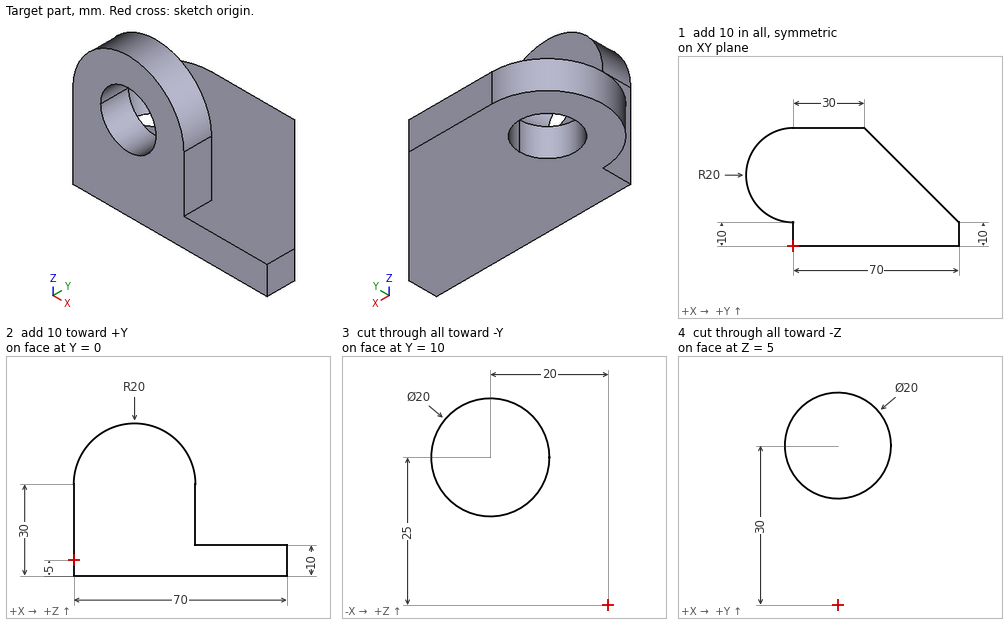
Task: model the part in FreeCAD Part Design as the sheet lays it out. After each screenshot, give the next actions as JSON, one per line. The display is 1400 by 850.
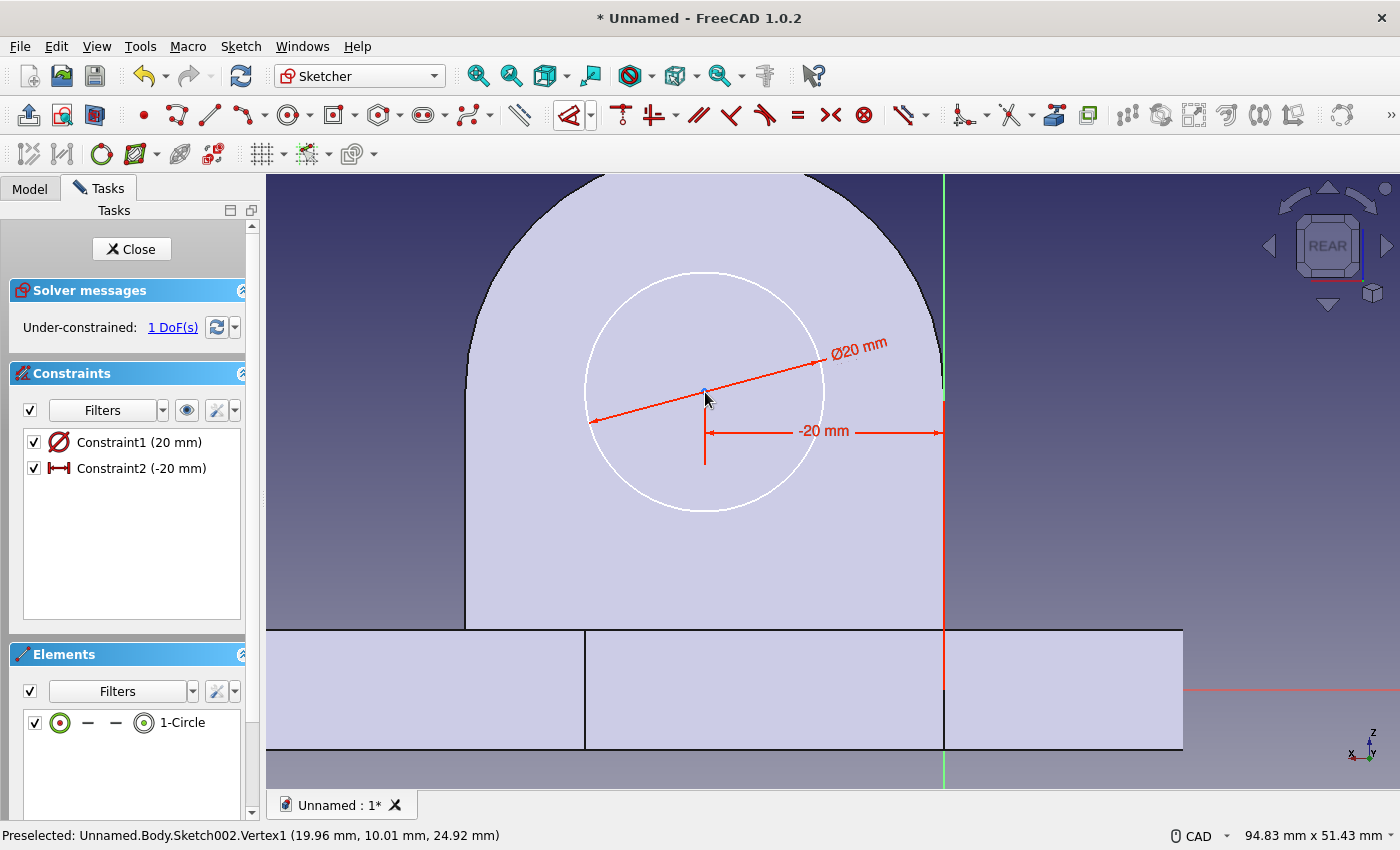
{"action": "left_click", "coordinate": [705, 392]}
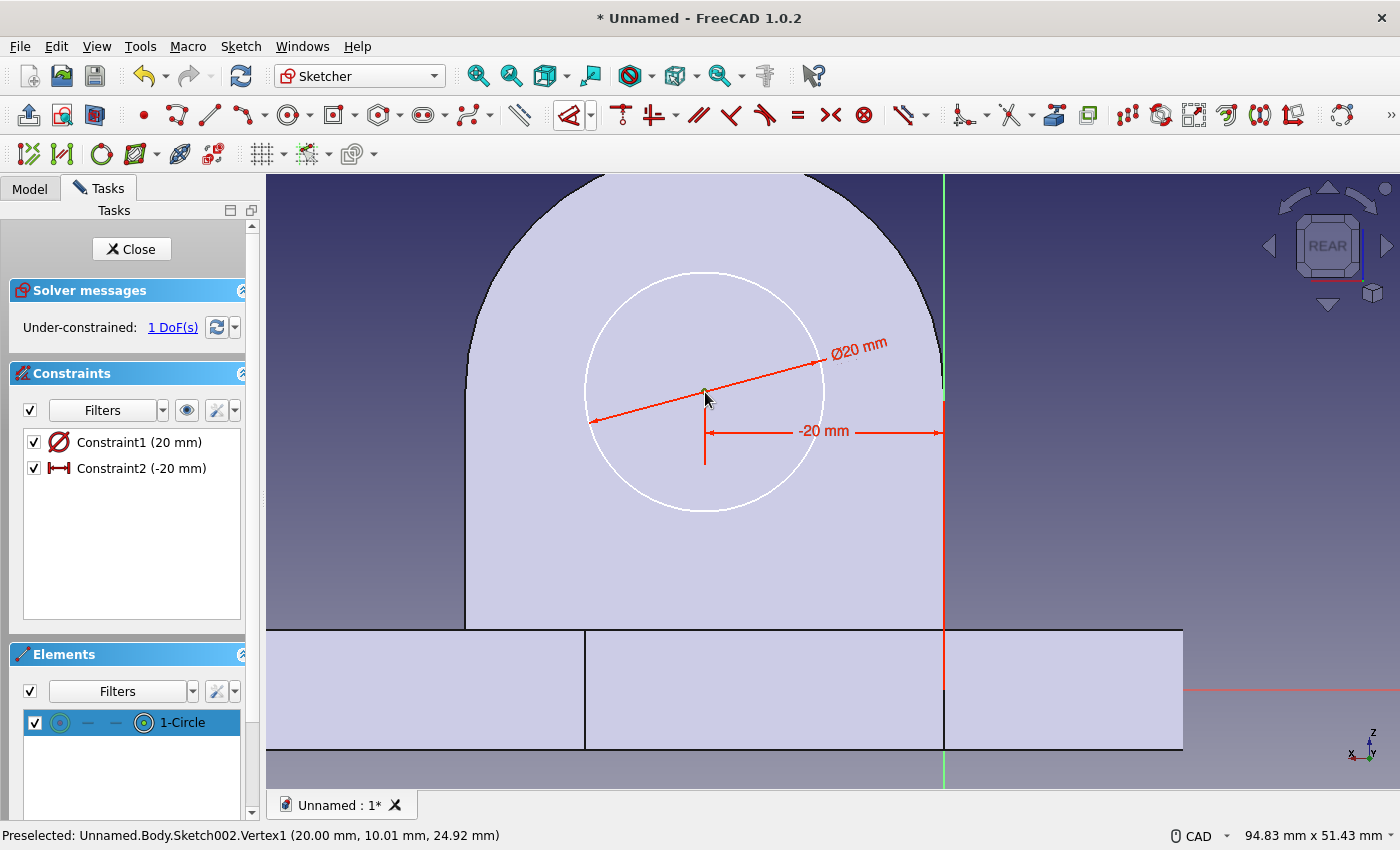
{"action": "key", "text": "i"}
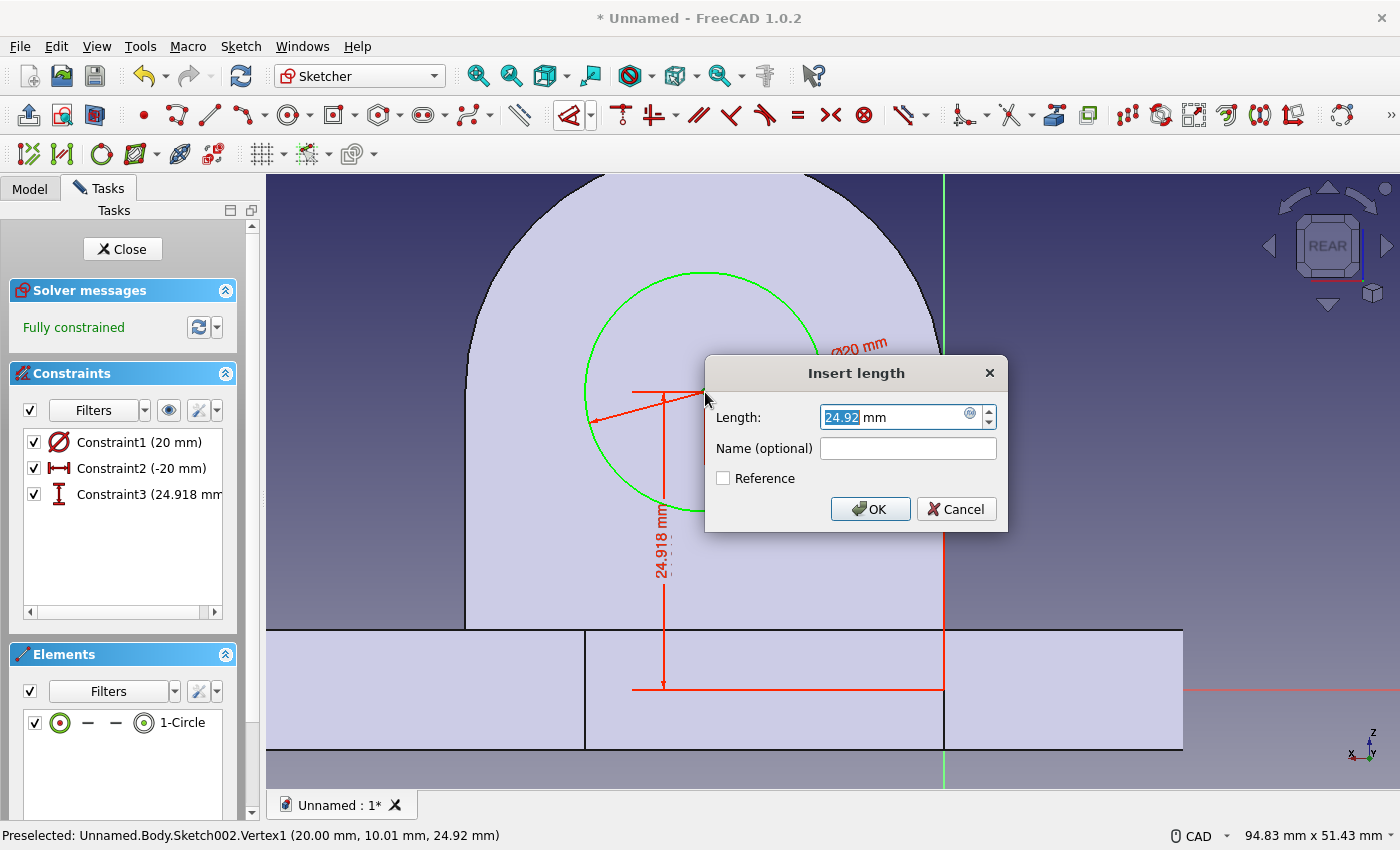
{"action": "type", "text": "25"}
{"action": "key", "text": "Return"}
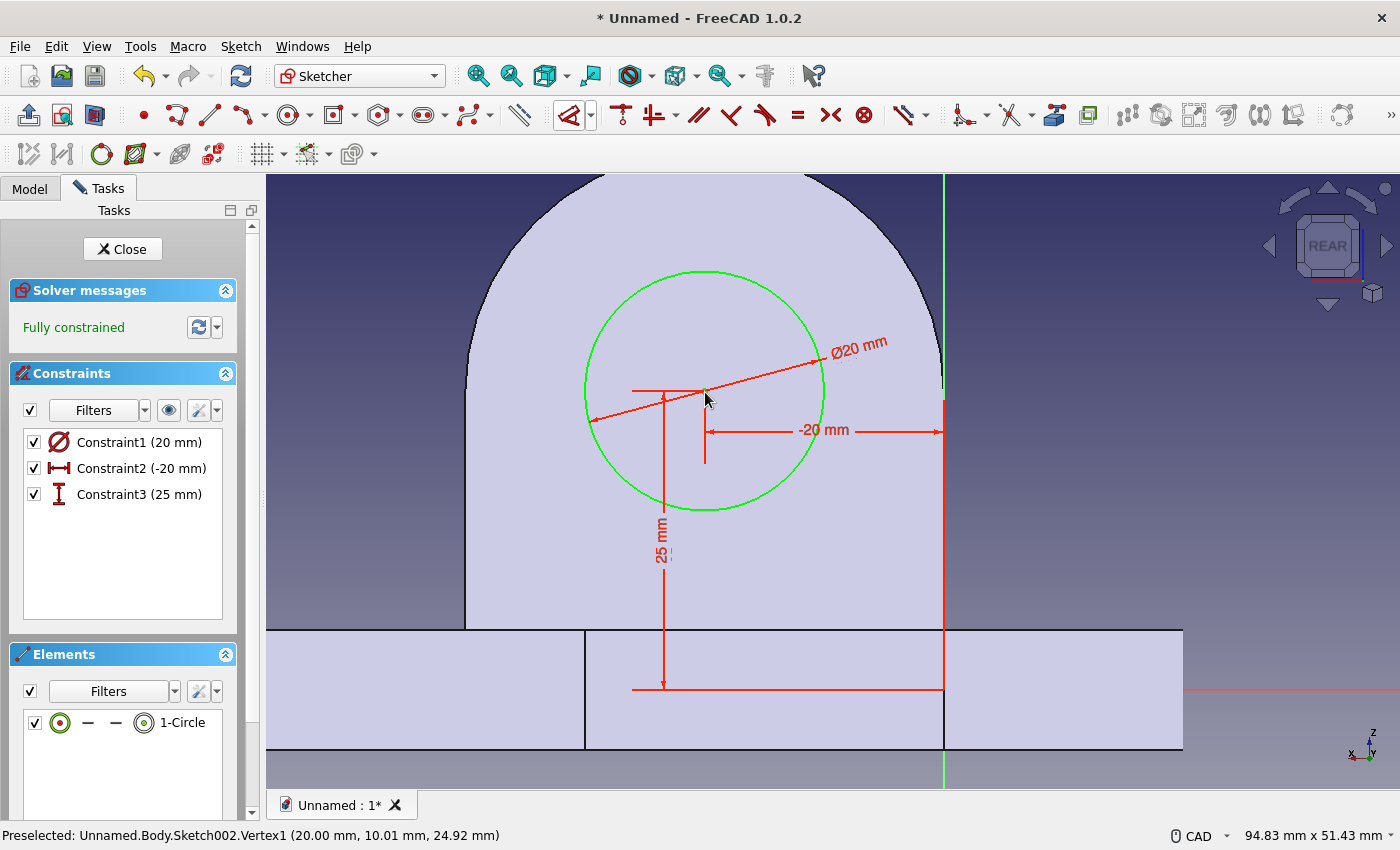
{"action": "left_click", "coordinate": [123, 249]}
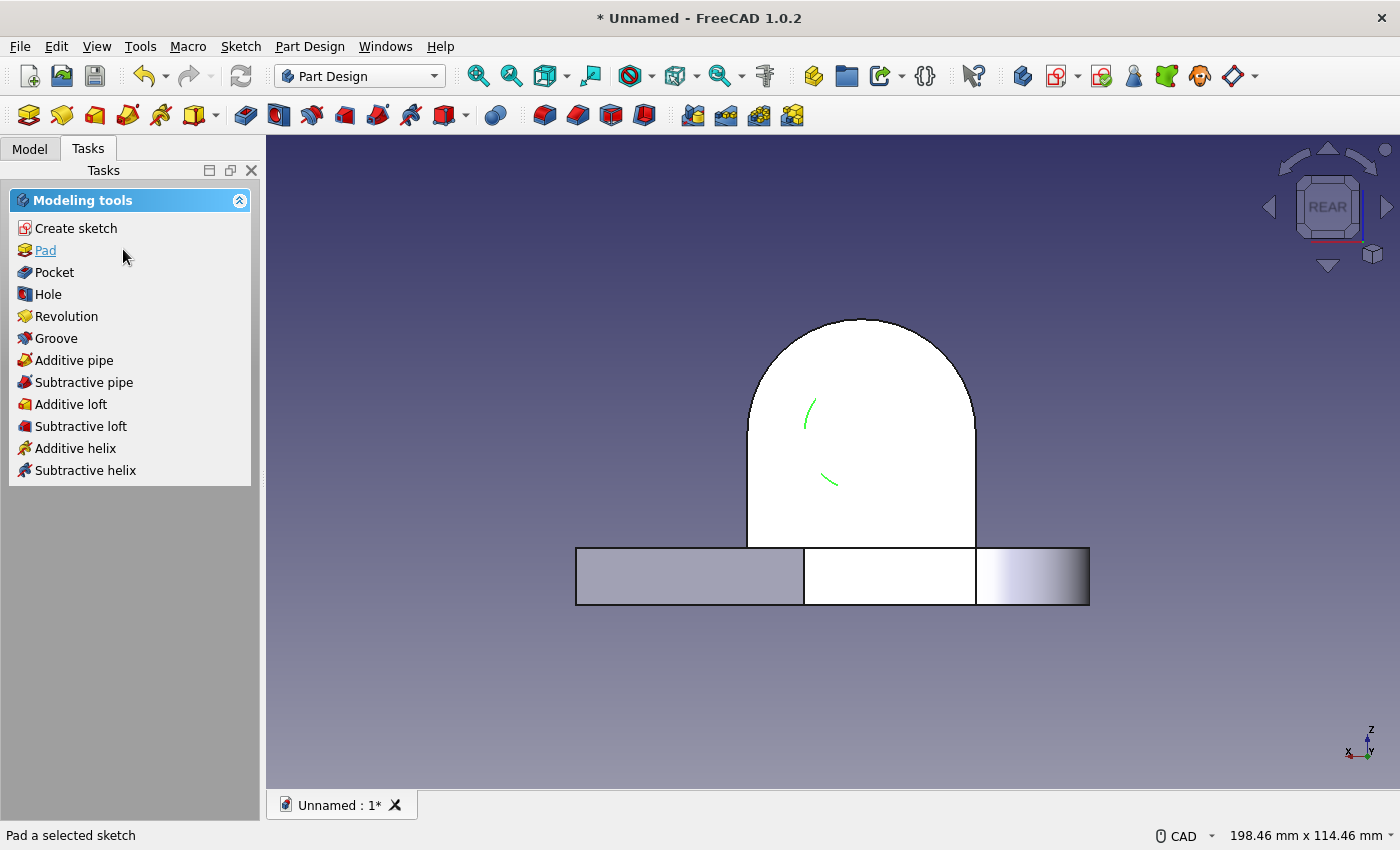
{"action": "left_click", "coordinate": [246, 116]}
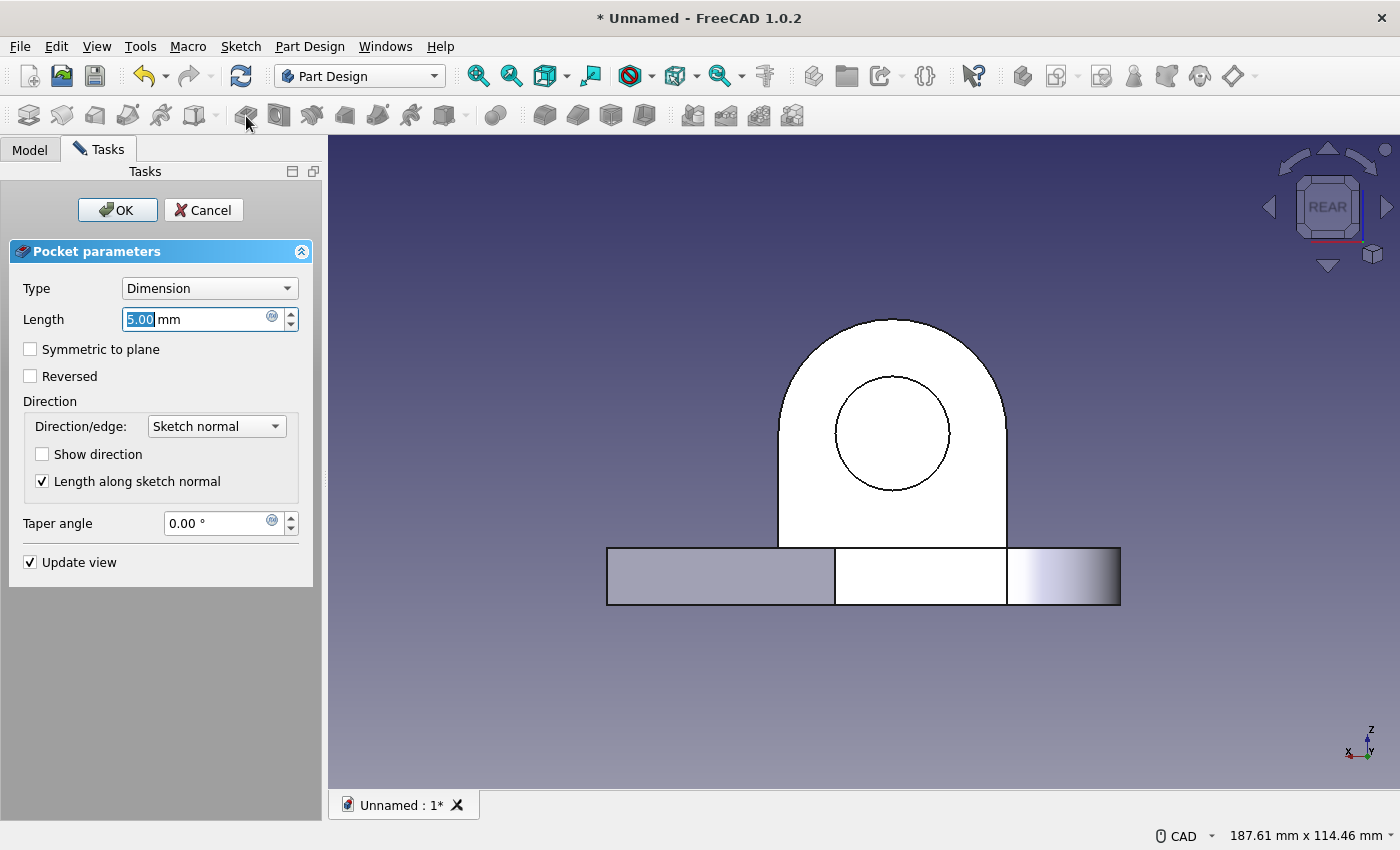
{"action": "left_click", "coordinate": [210, 288]}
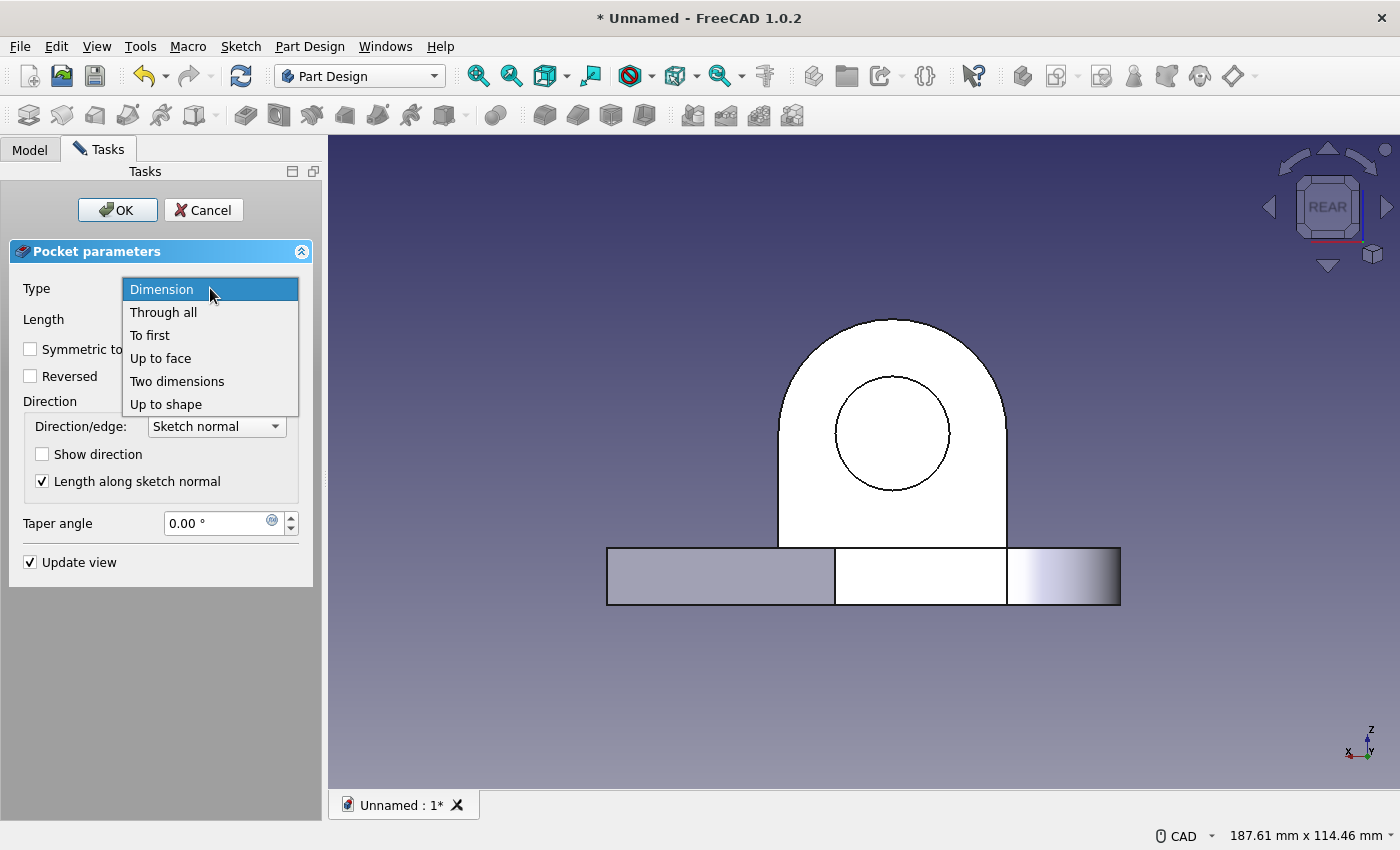
{"action": "left_click", "coordinate": [208, 312]}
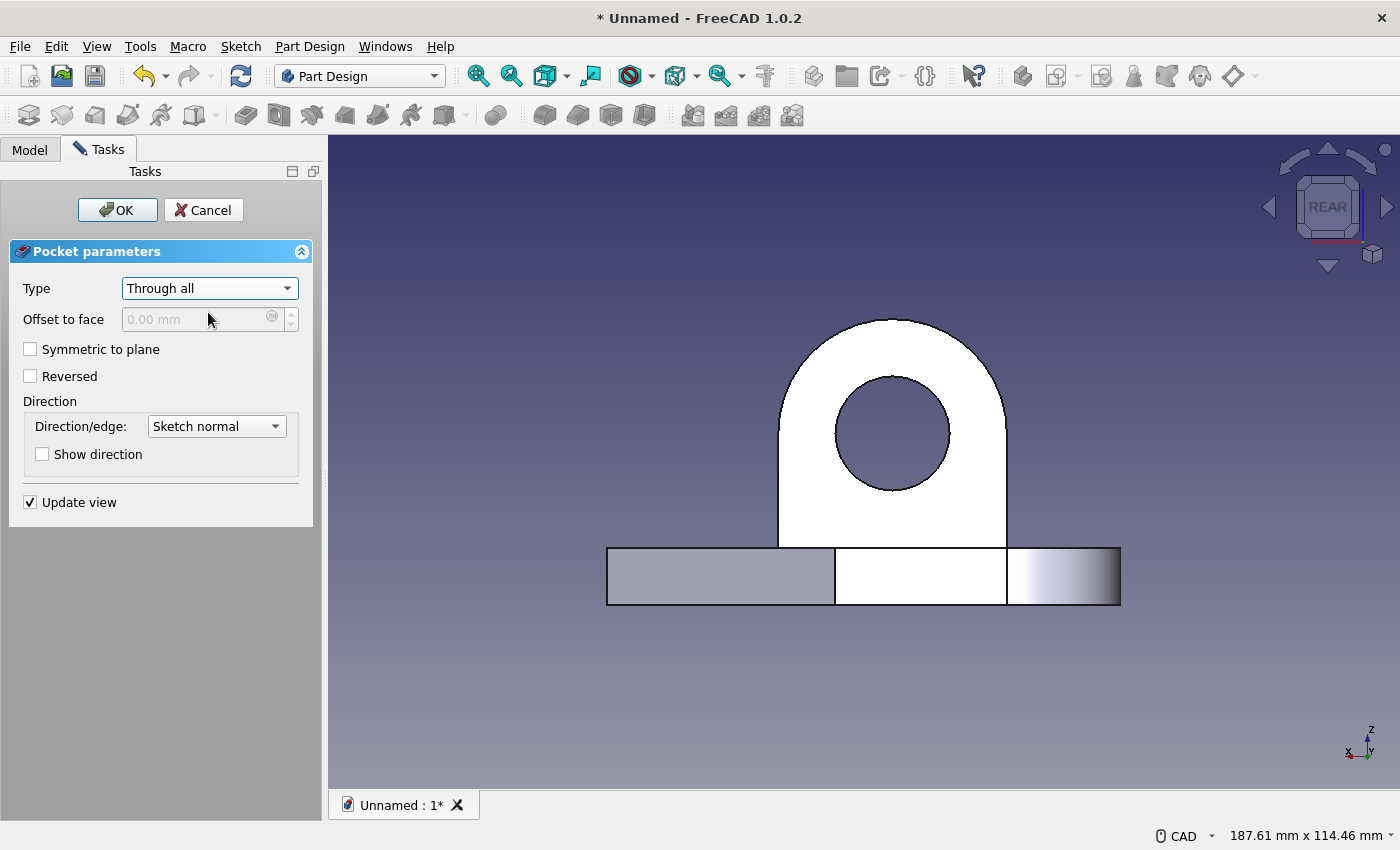
{"action": "left_click", "coordinate": [118, 210]}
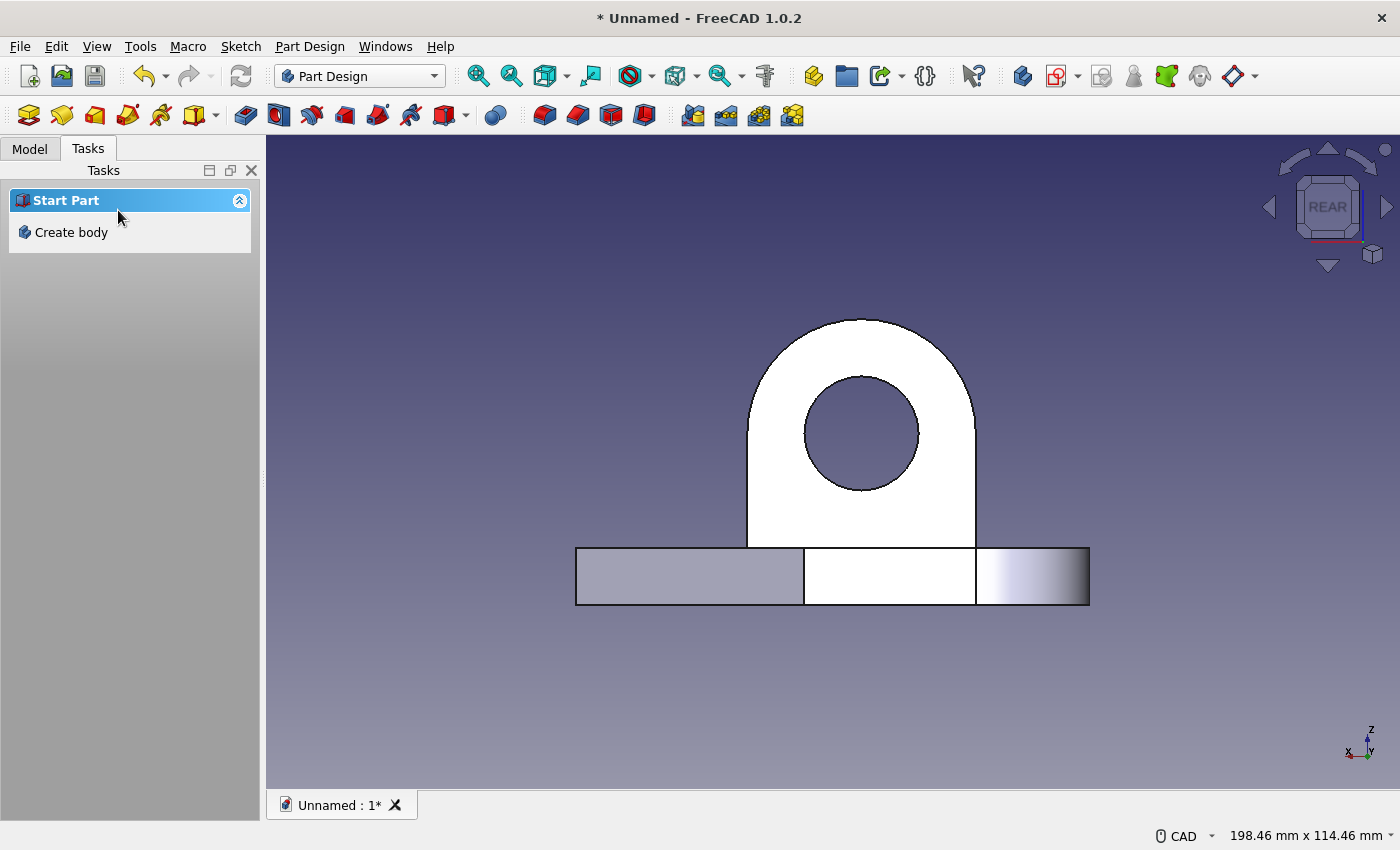
{"action": "key", "text": "0"}